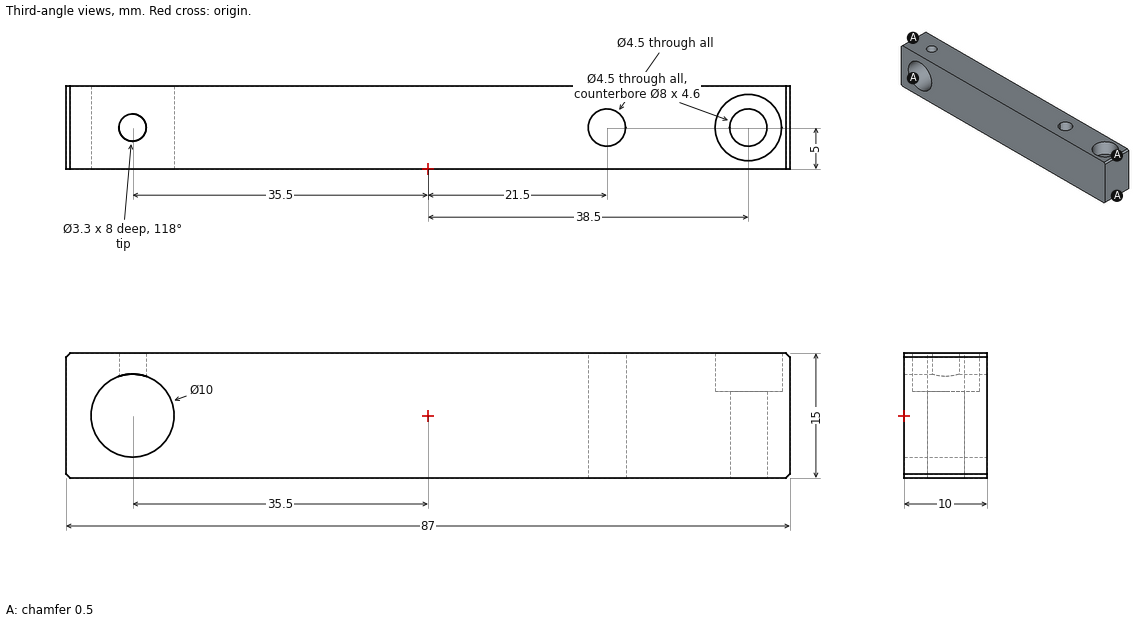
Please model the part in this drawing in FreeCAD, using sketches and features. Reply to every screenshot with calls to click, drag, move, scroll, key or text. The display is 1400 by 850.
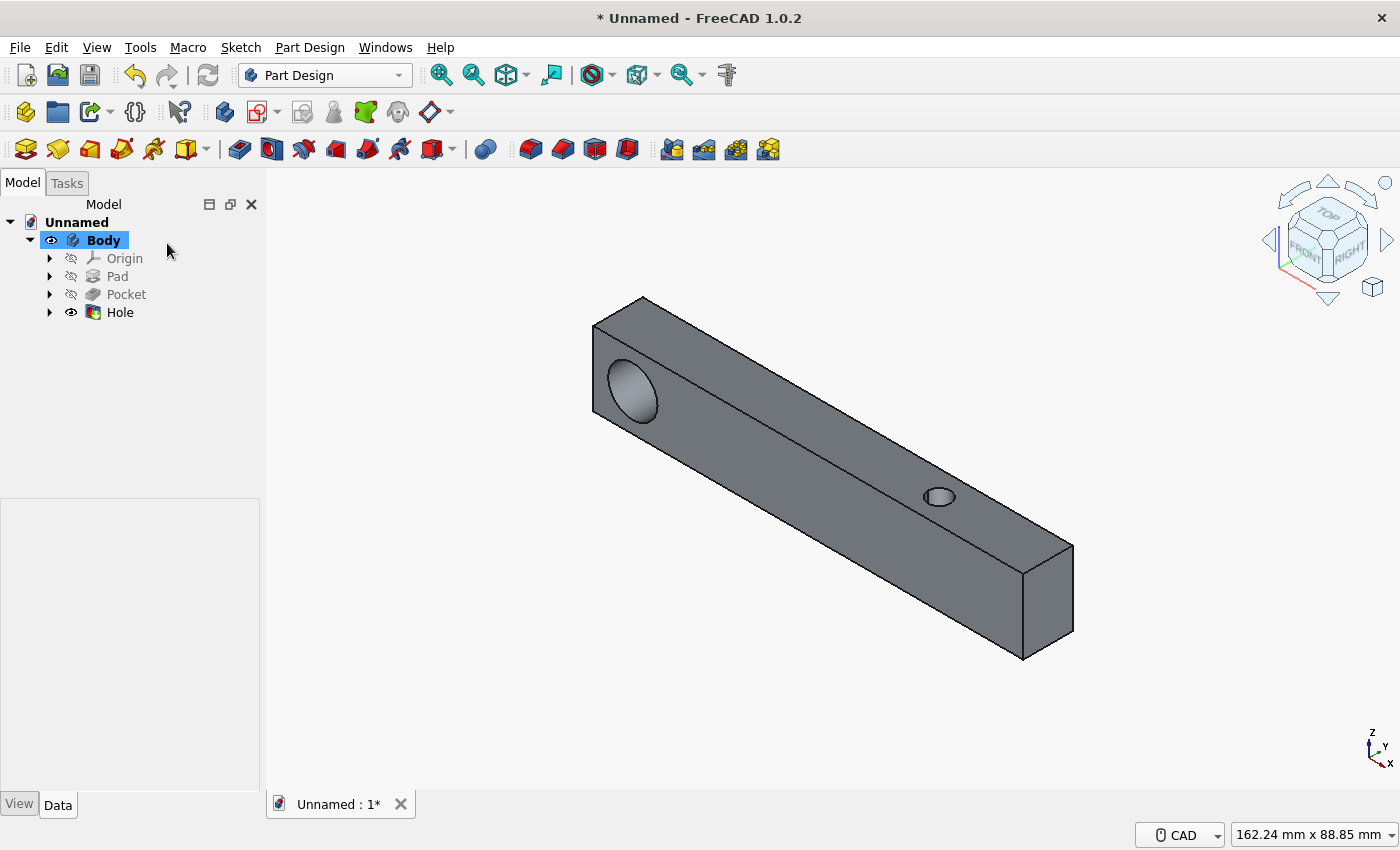
click(1017, 541)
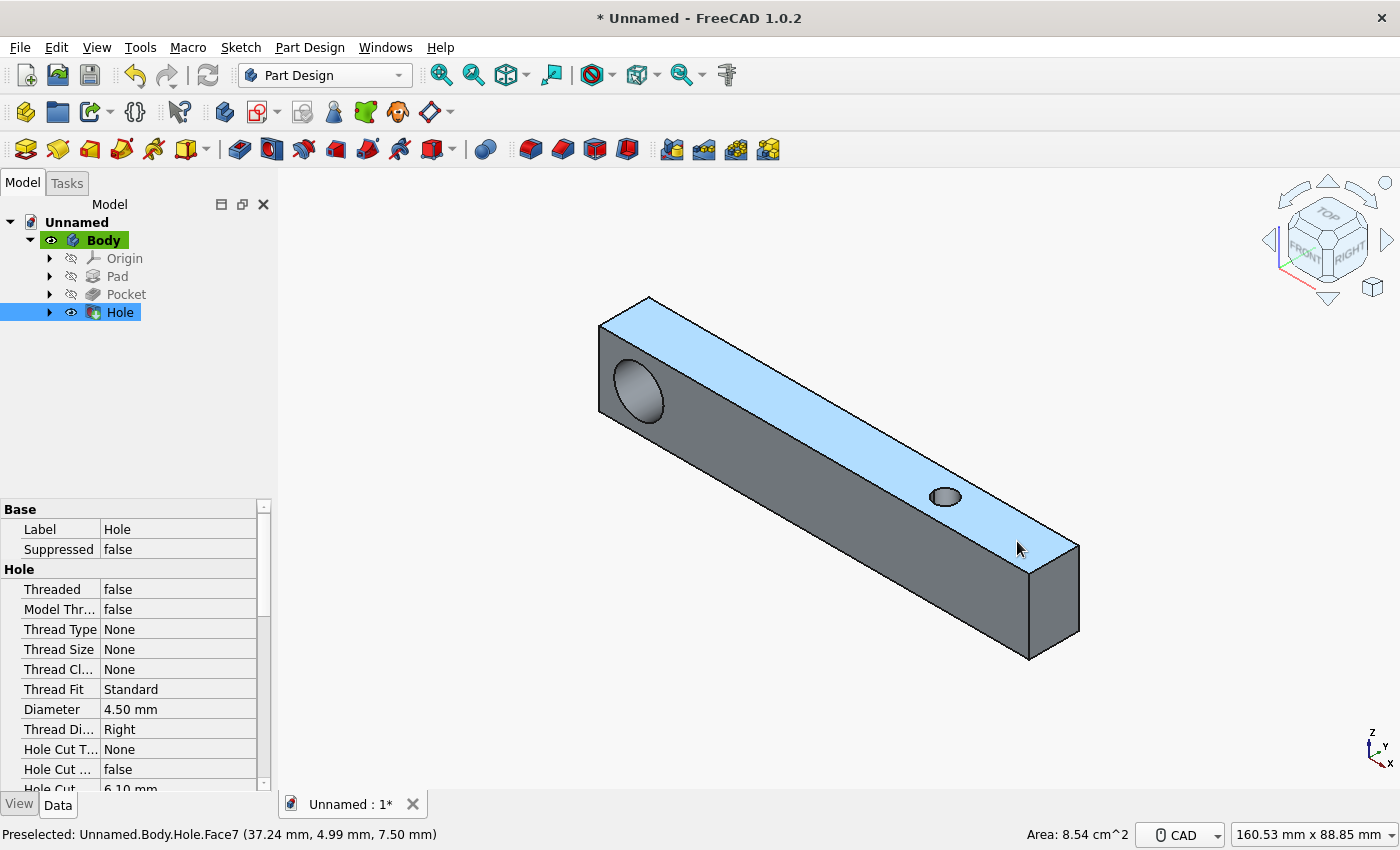
click(258, 112)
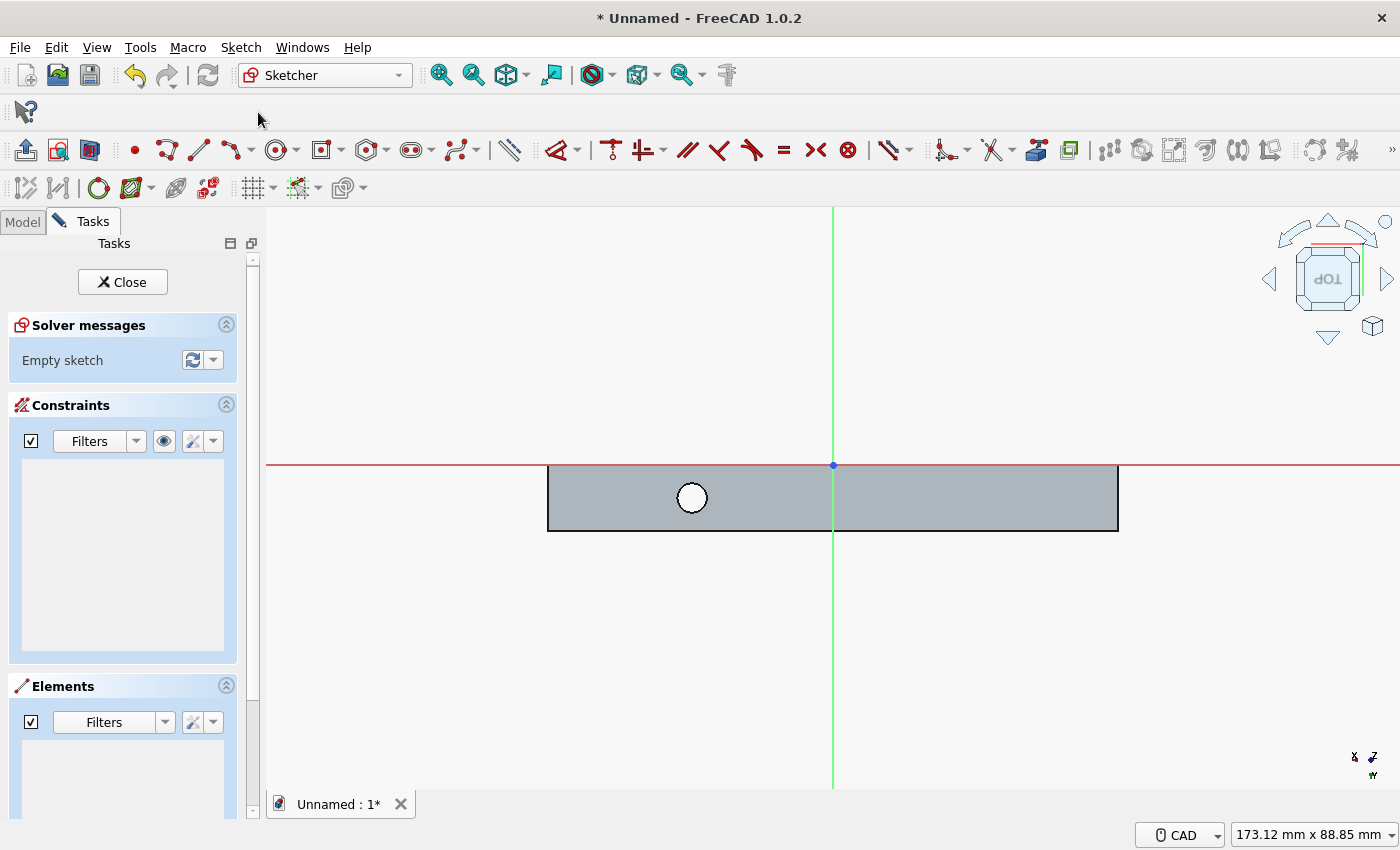
scroll(566, 498, up, 13)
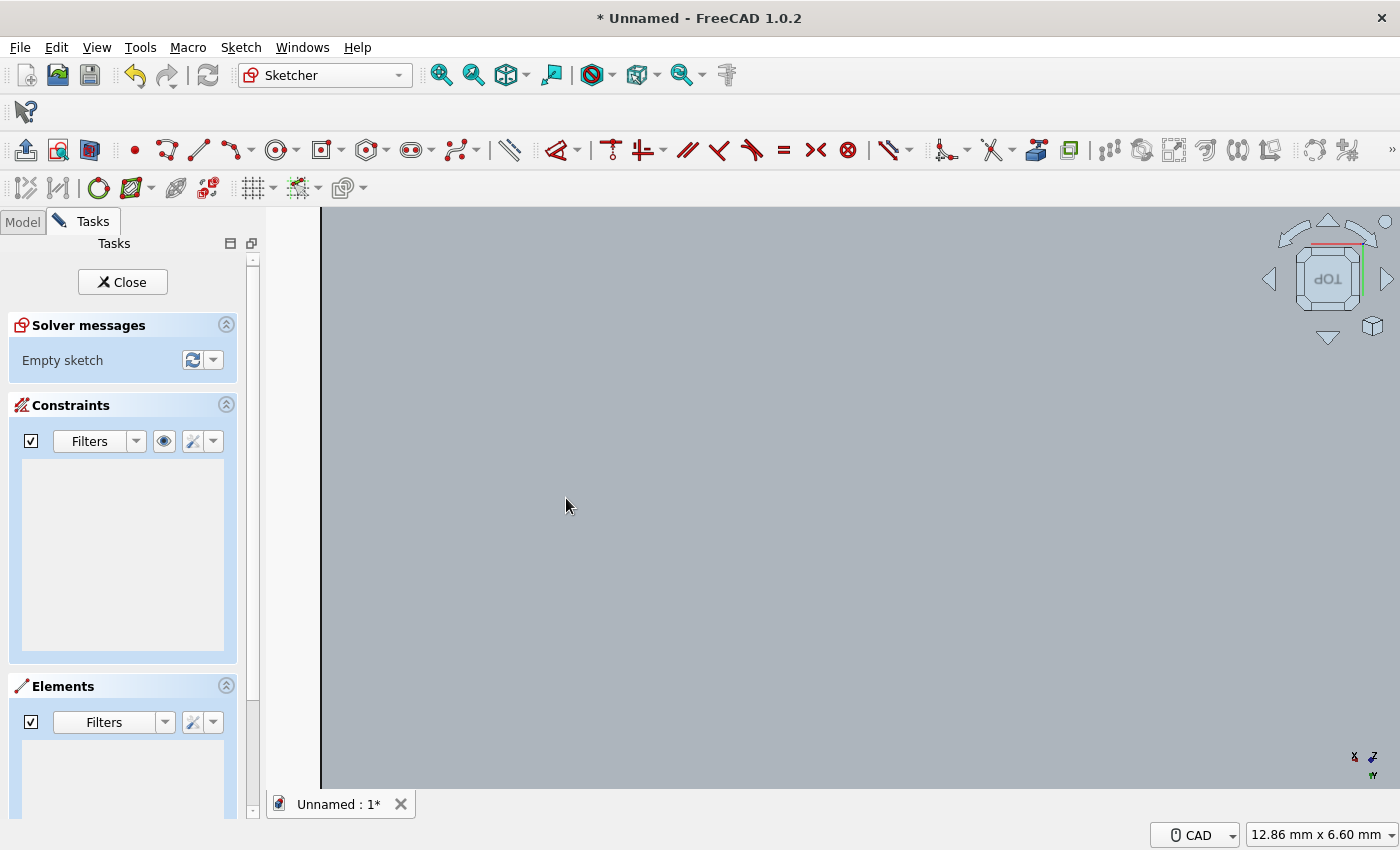
click(276, 150)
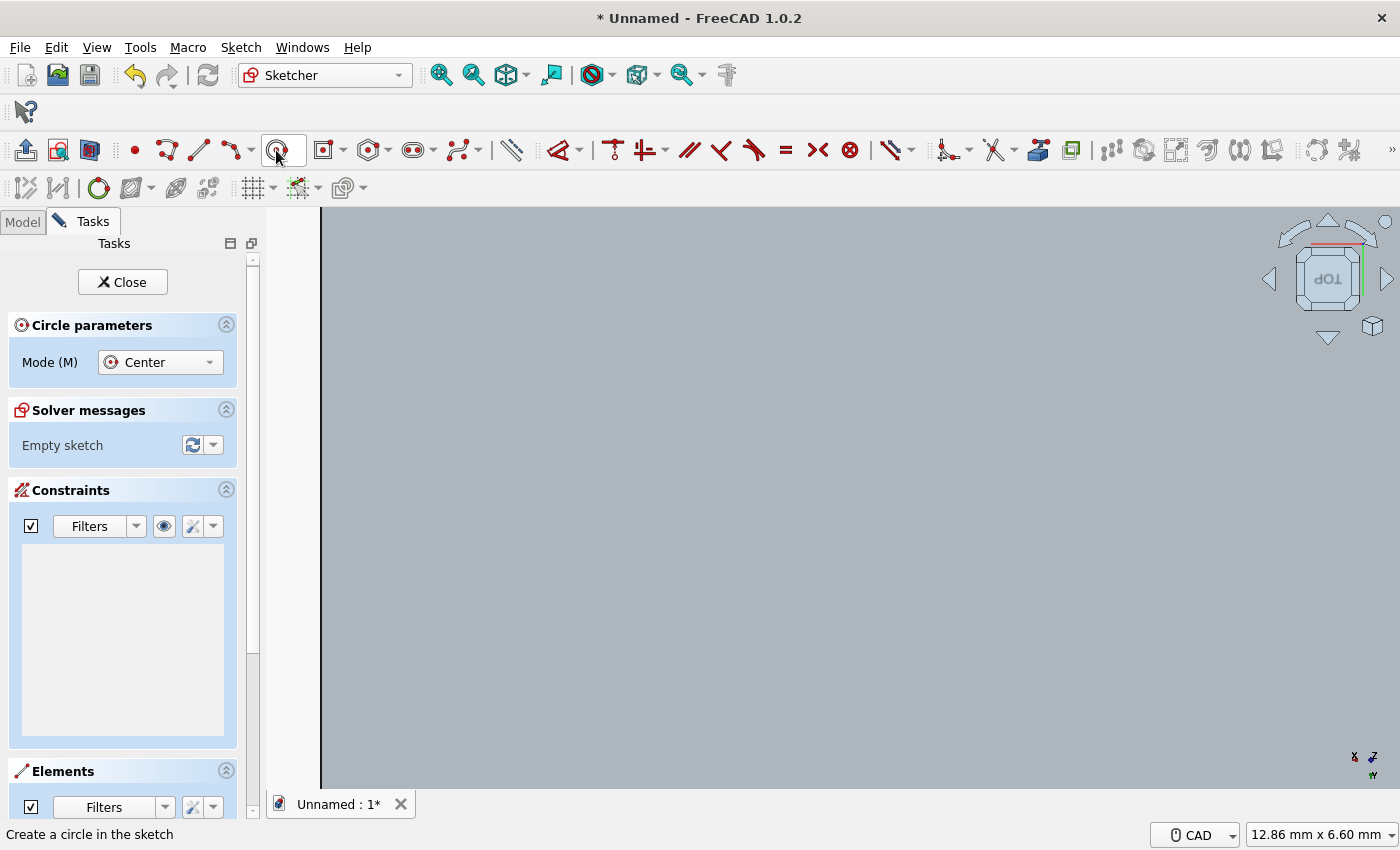
click(762, 492)
click(902, 351)
key(Escape)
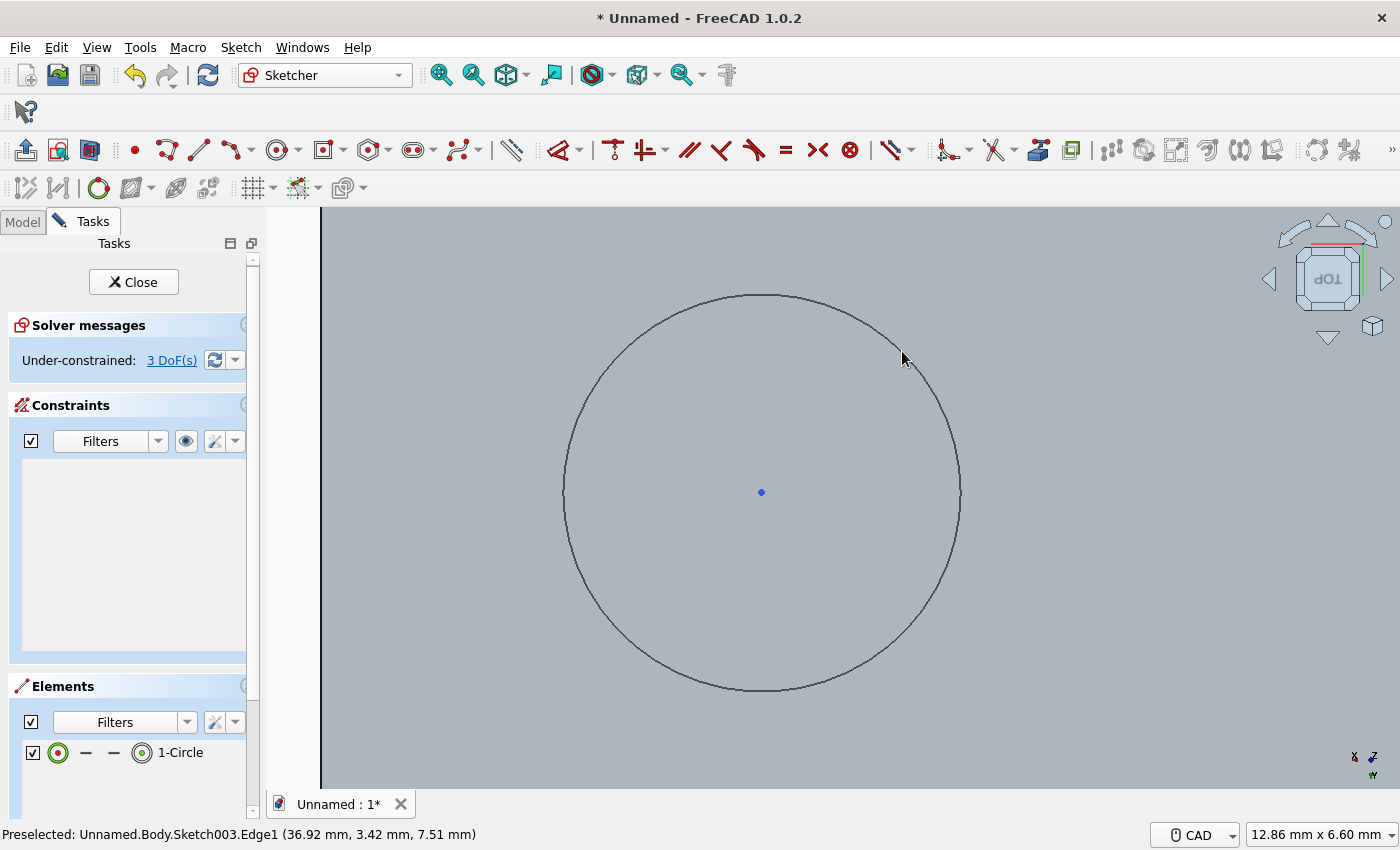
click(558, 150)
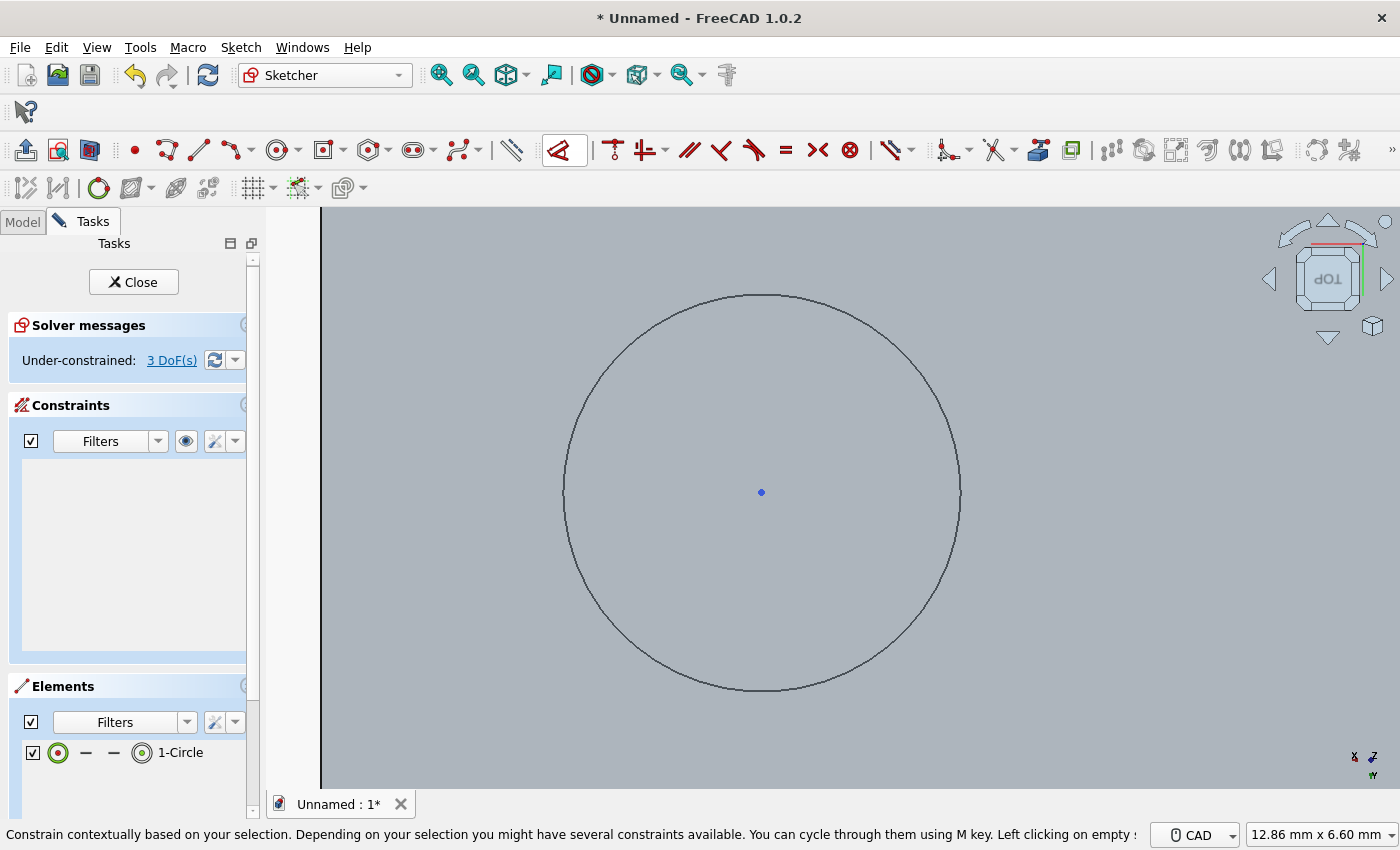
click(902, 352)
click(925, 329)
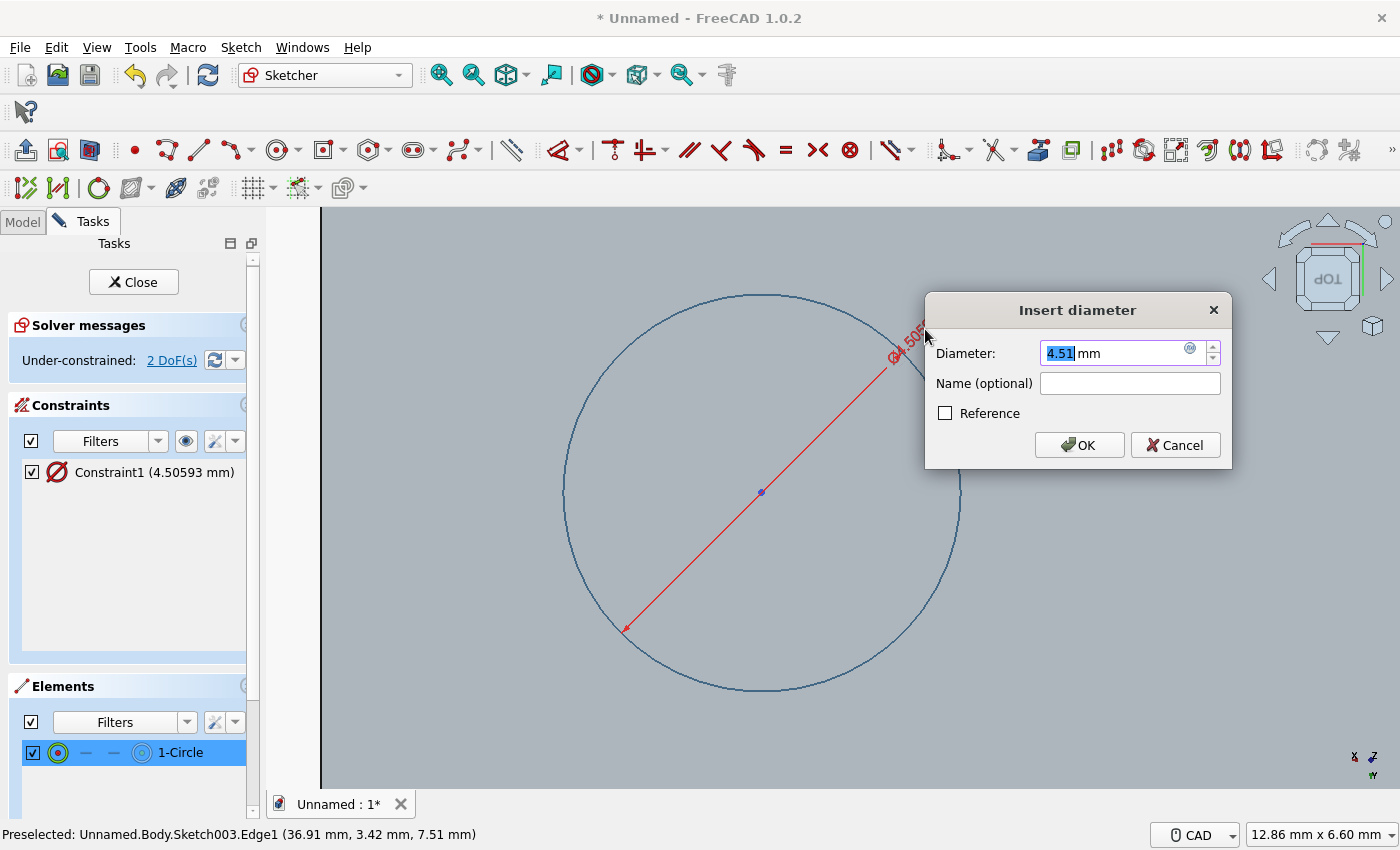
text(4.5)
key(Return)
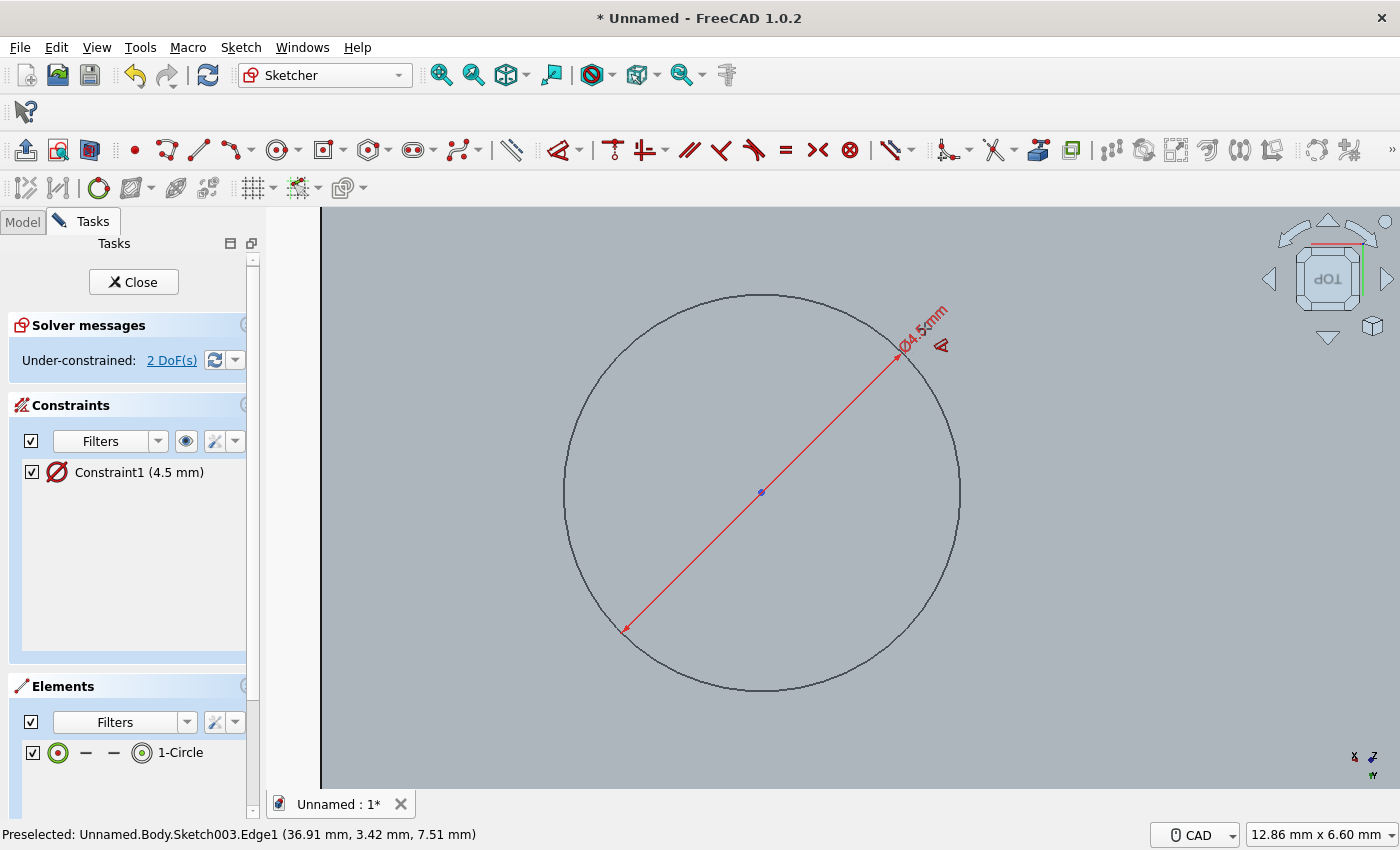
click(762, 493)
click(728, 364)